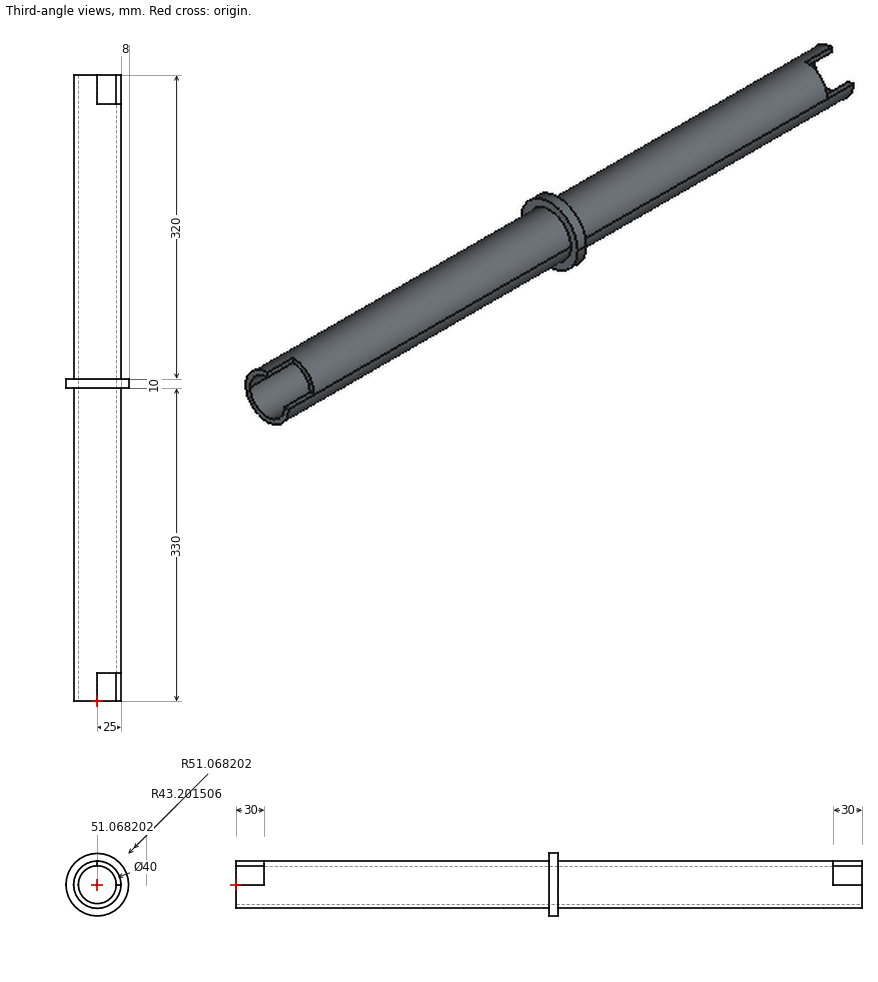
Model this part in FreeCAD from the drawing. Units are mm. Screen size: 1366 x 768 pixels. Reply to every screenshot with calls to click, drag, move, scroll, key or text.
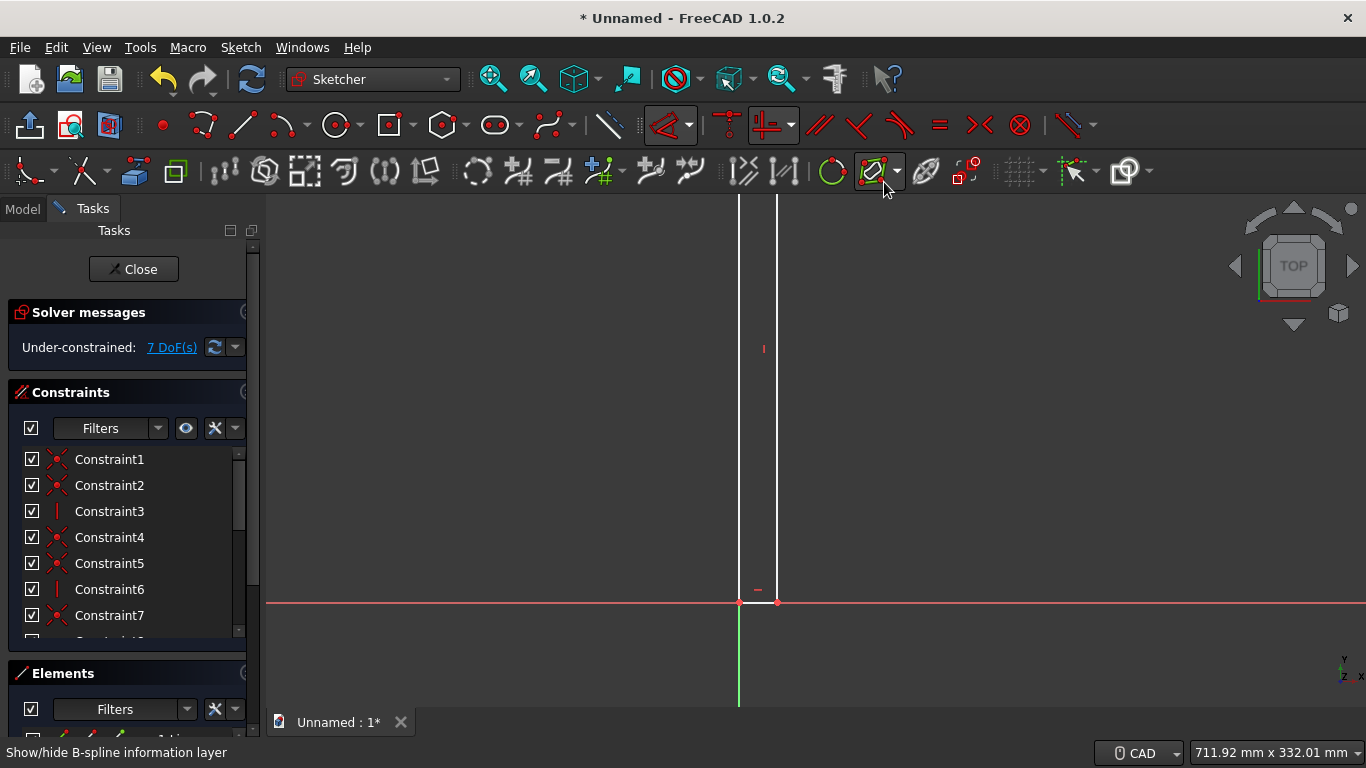
scroll(740, 605, down, 6)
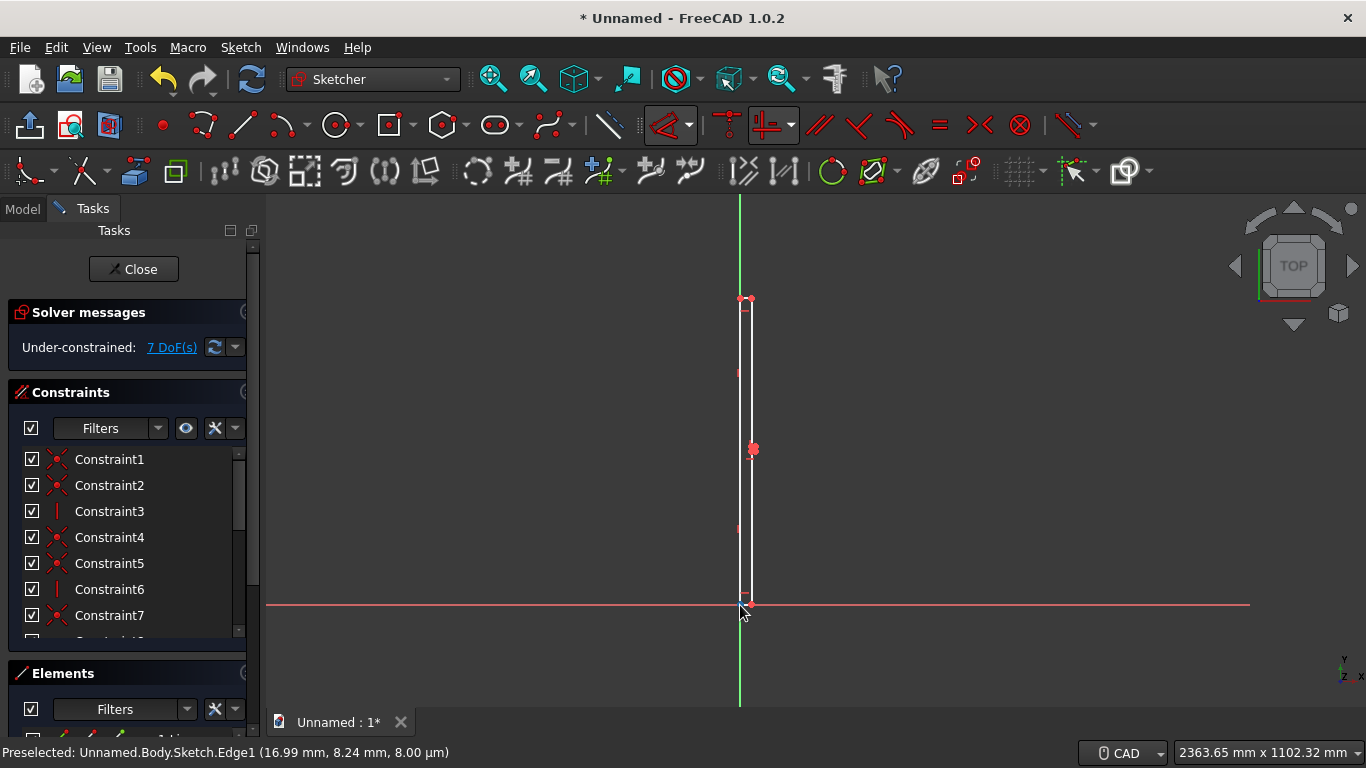
scroll(753, 452, up, 10)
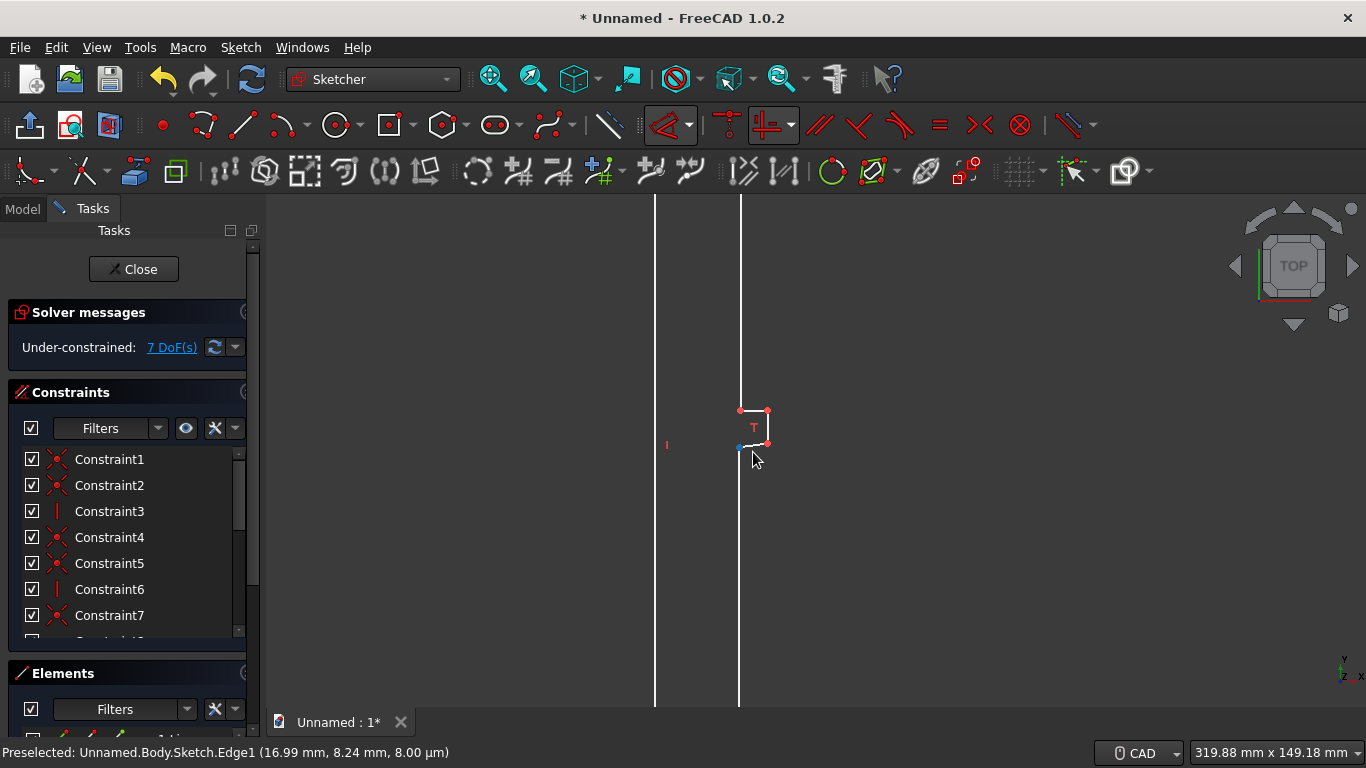
click(753, 445)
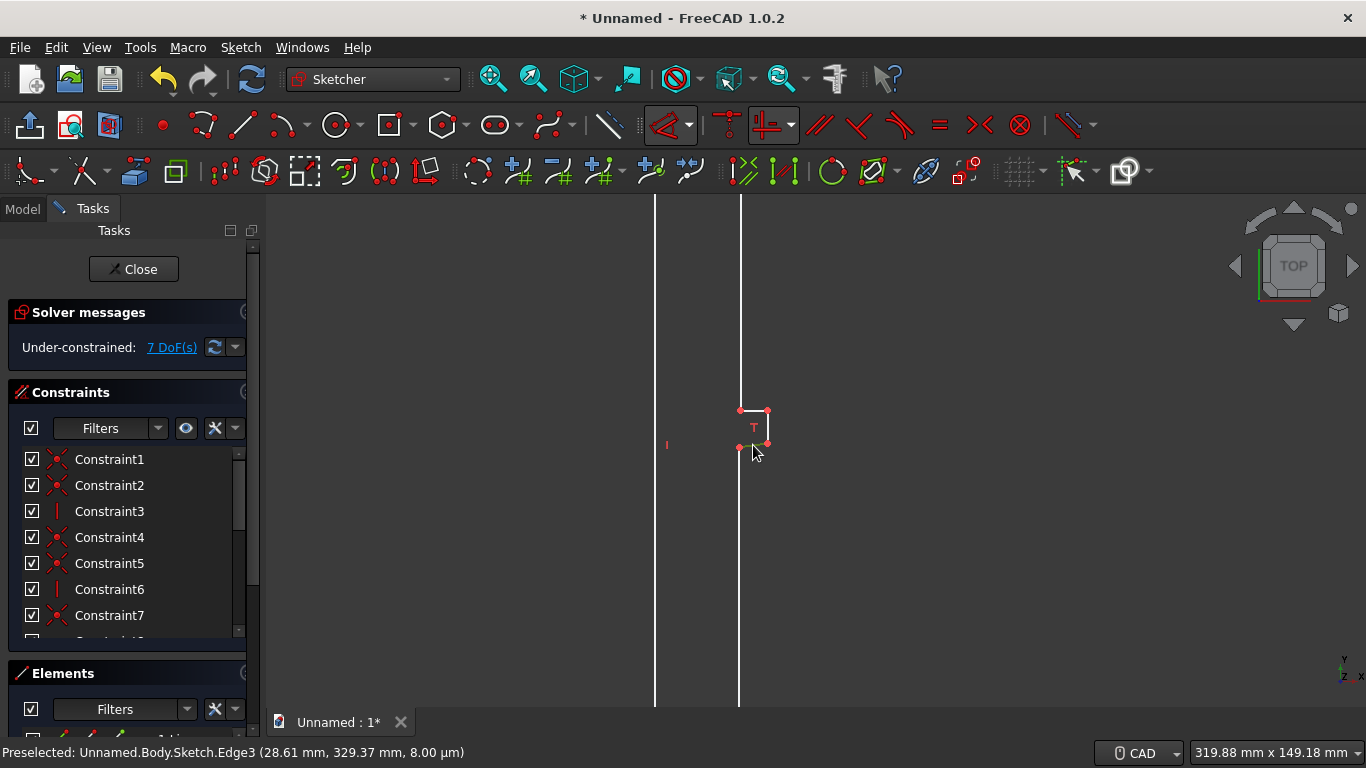
key(h)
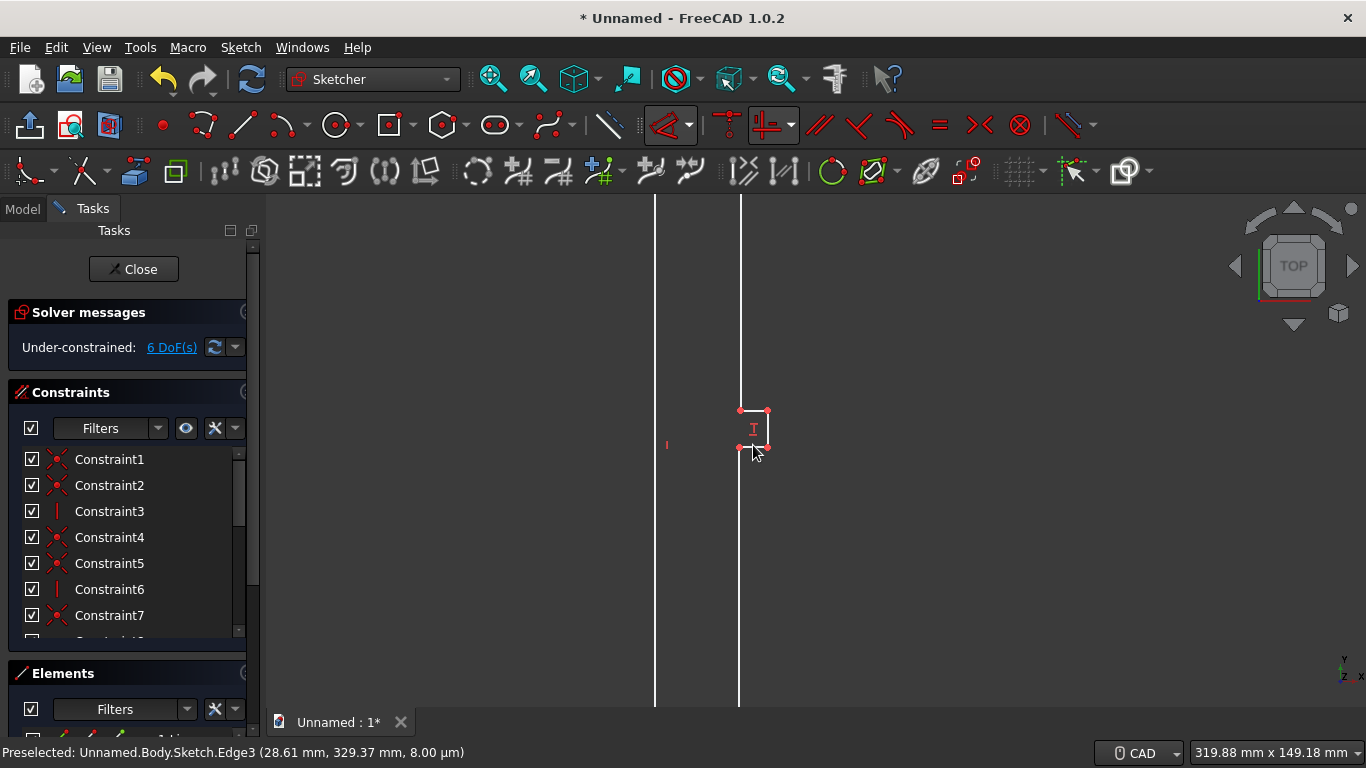
click(664, 126)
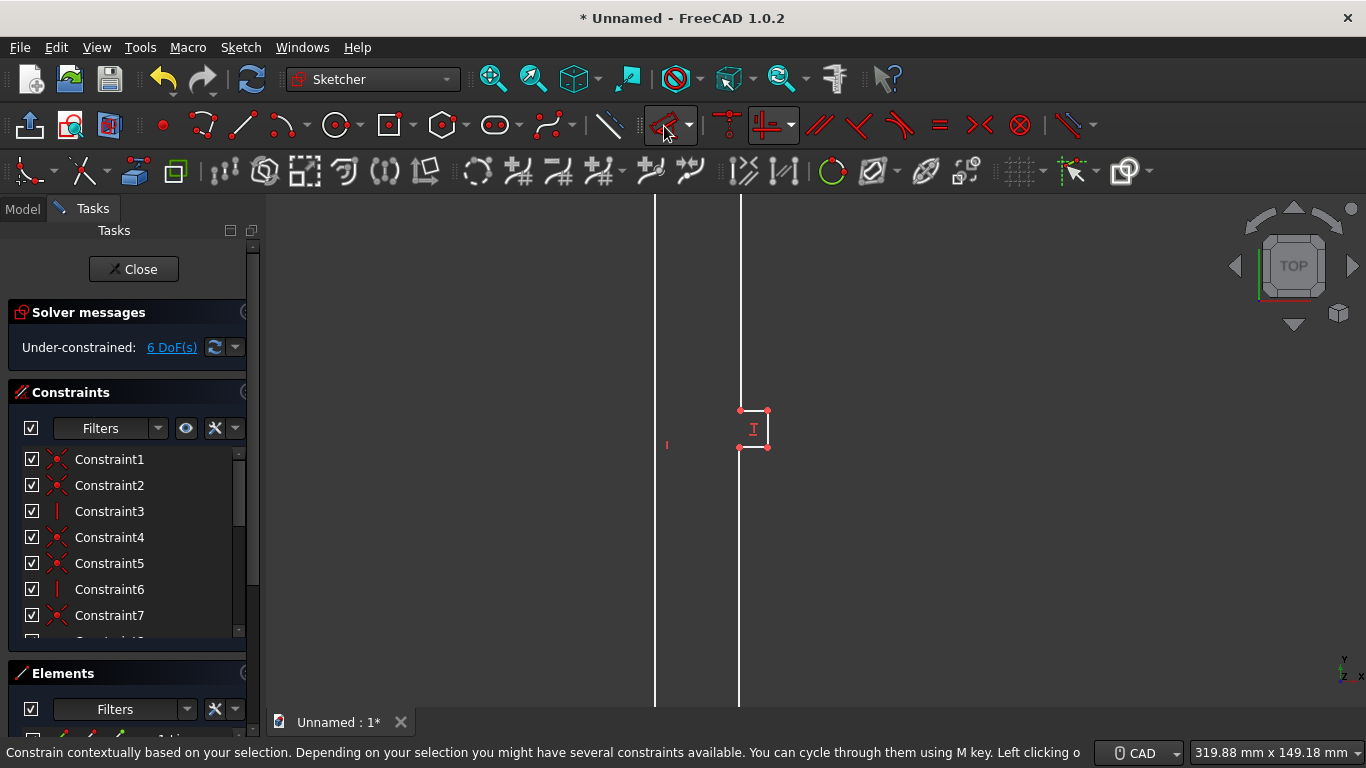
scroll(751, 447, up, 2)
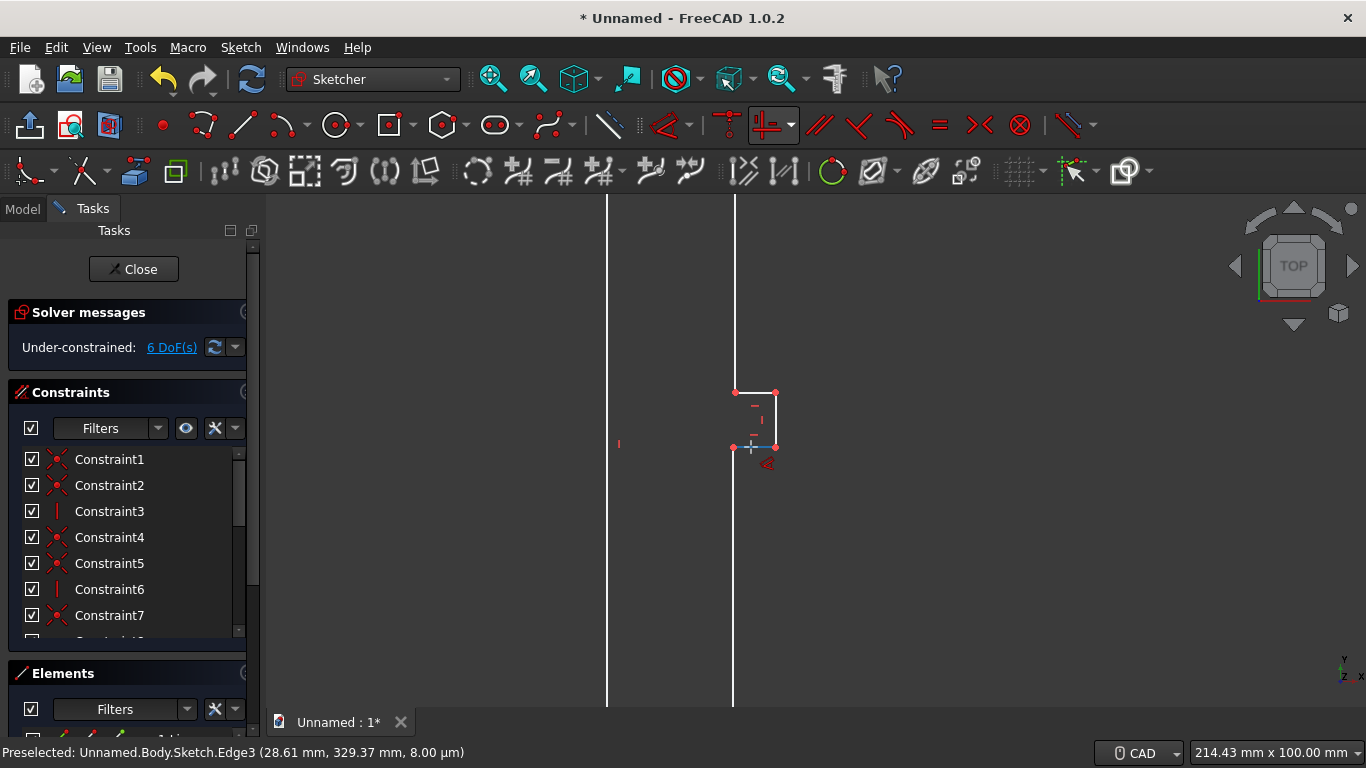
click(750, 447)
click(754, 481)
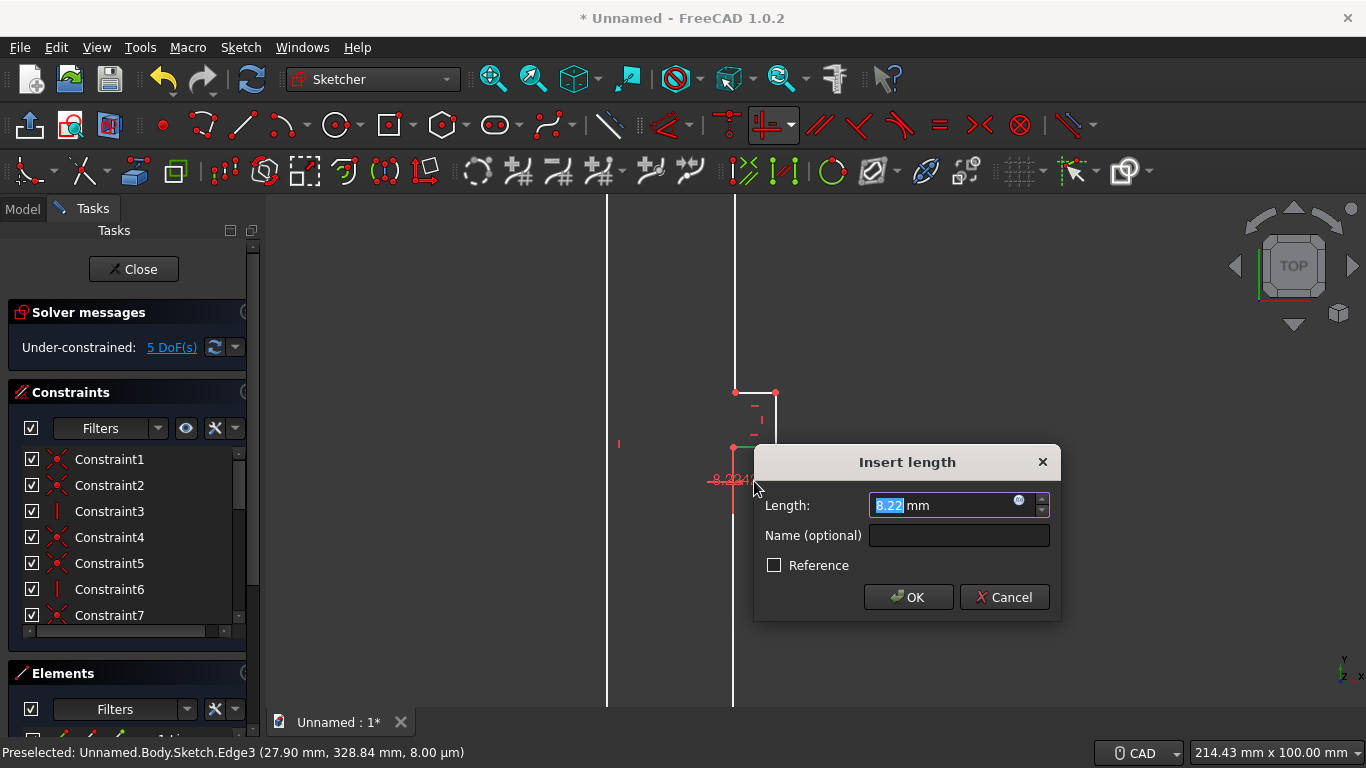
text(8)
key(Return)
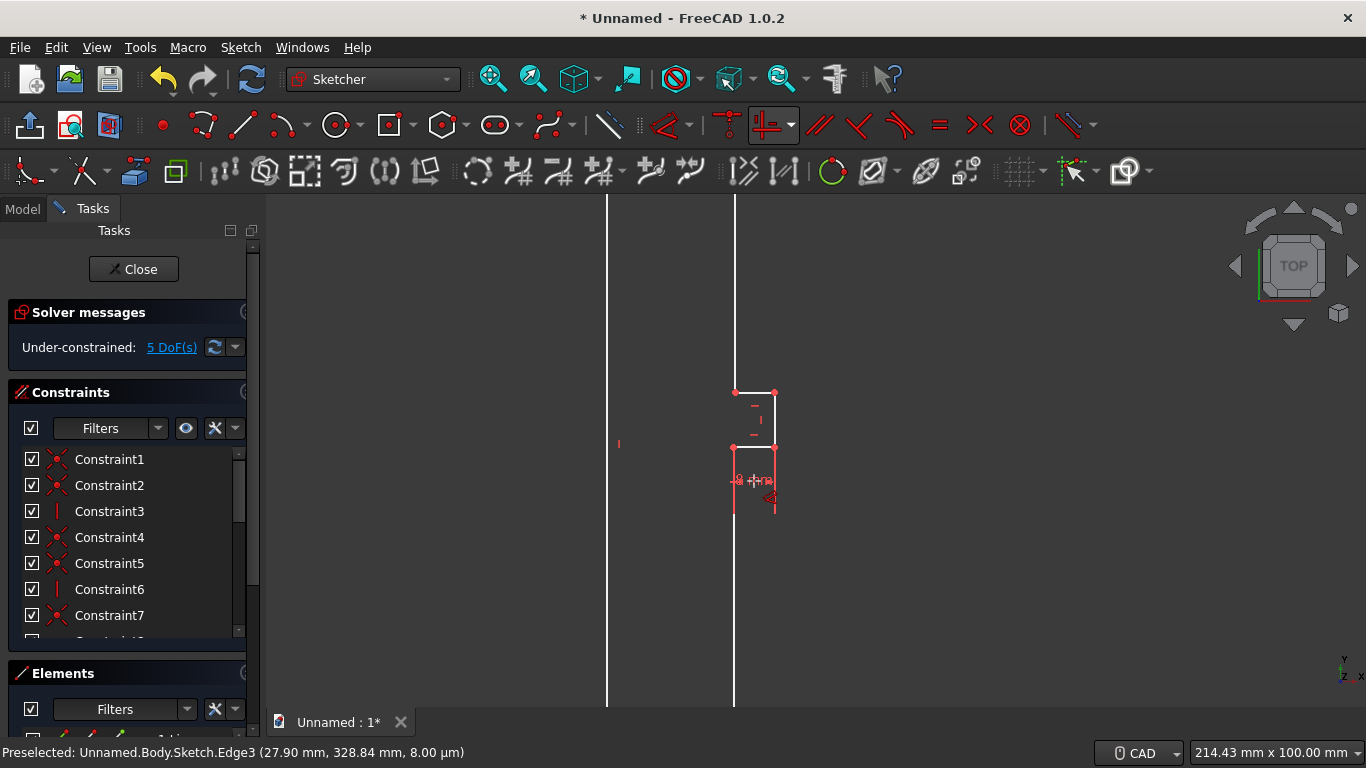
click(763, 393)
click(755, 359)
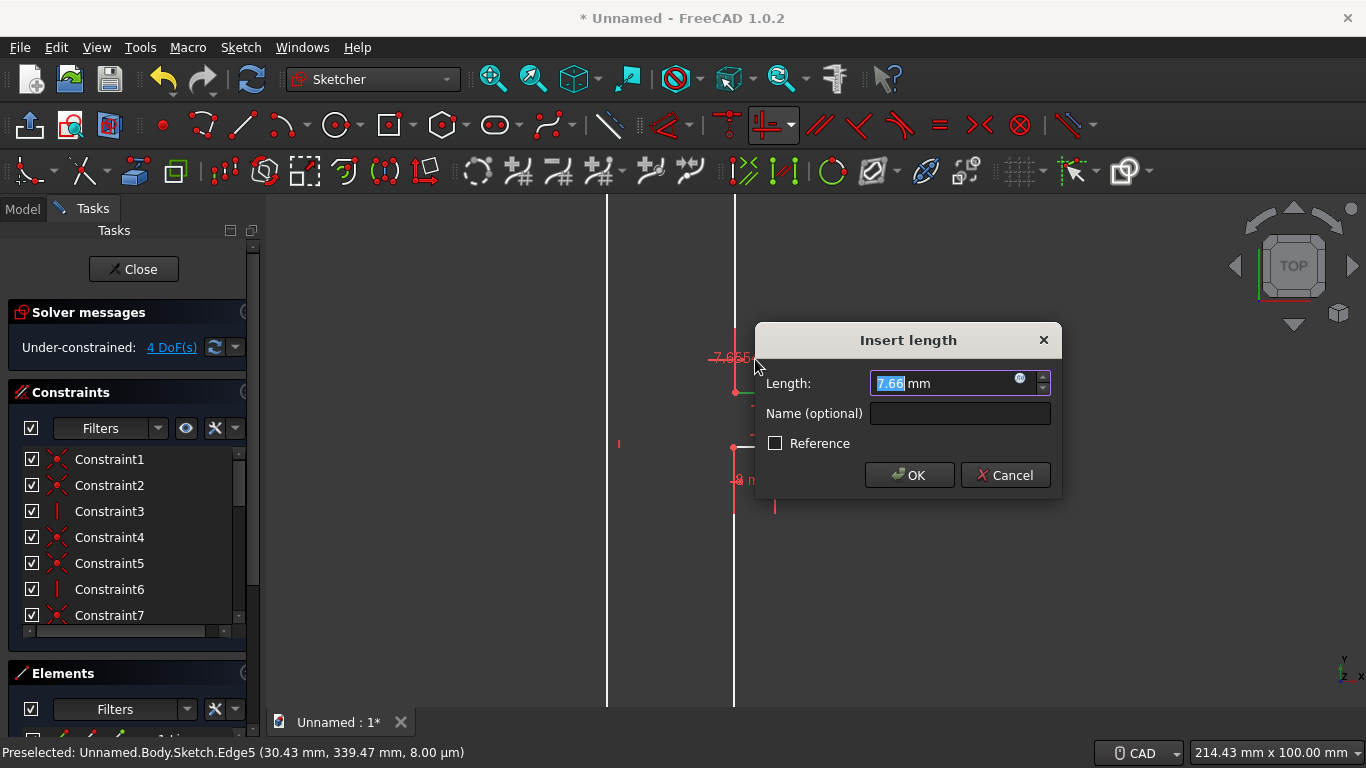
text(8)
key(Return)